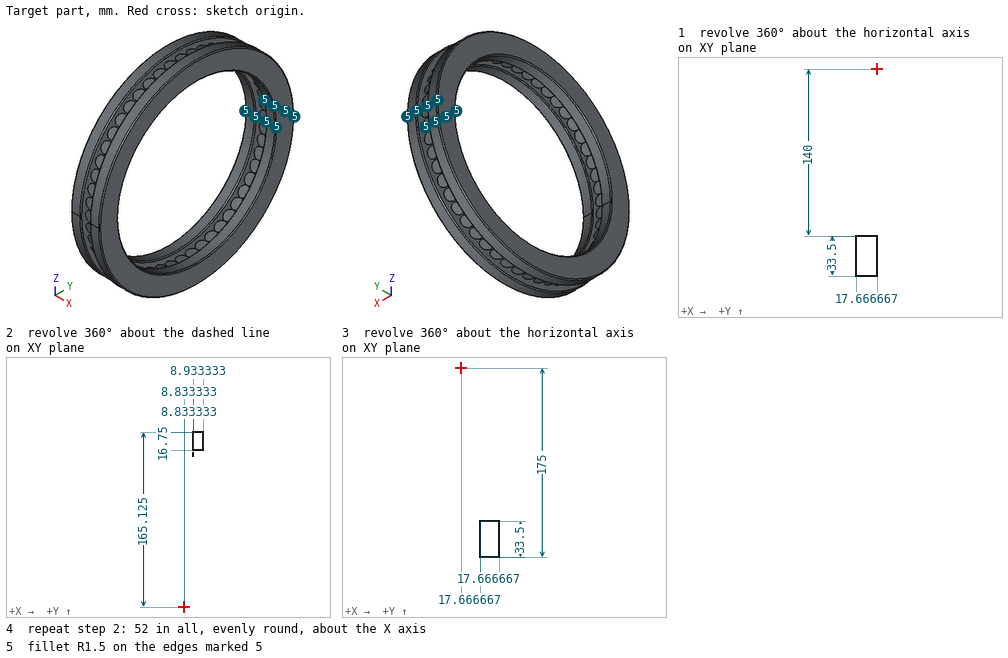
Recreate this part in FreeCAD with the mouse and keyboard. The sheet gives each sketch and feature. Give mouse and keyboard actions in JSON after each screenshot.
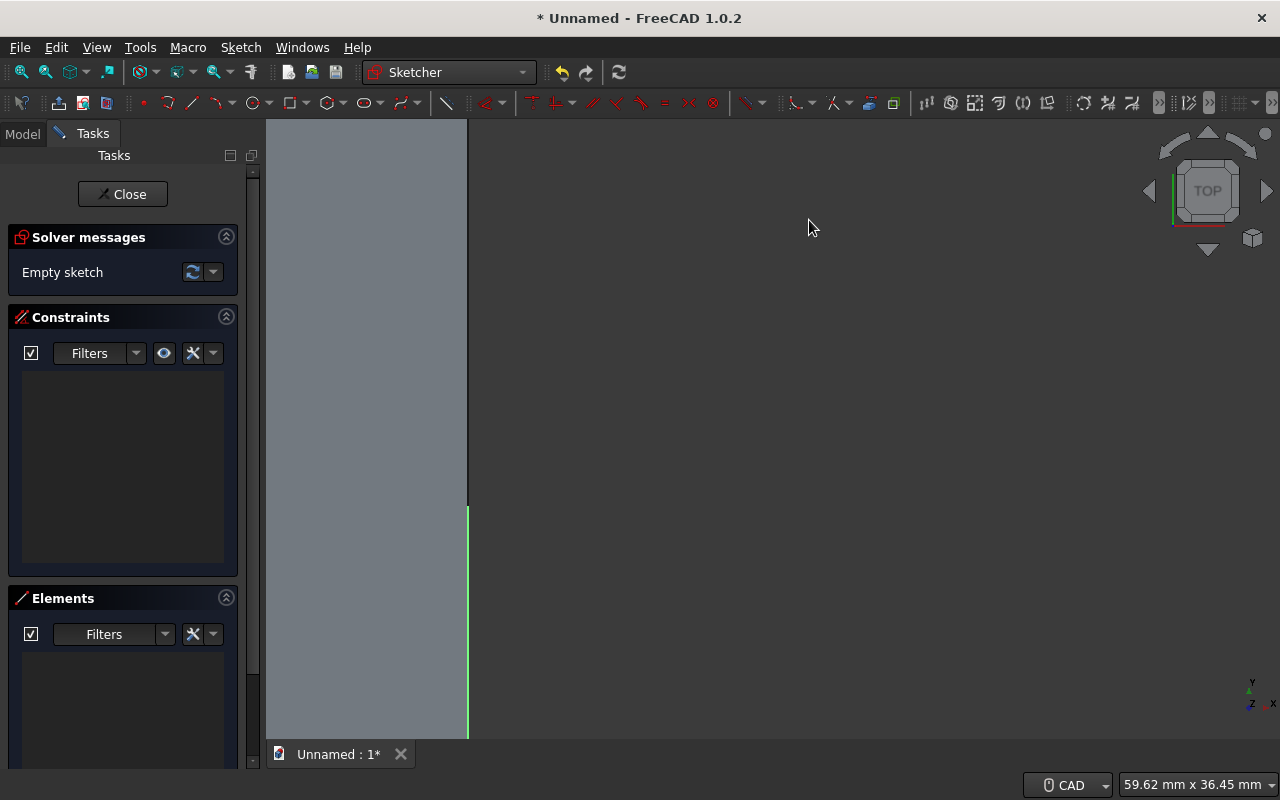
{"action": "key", "text": "g r"}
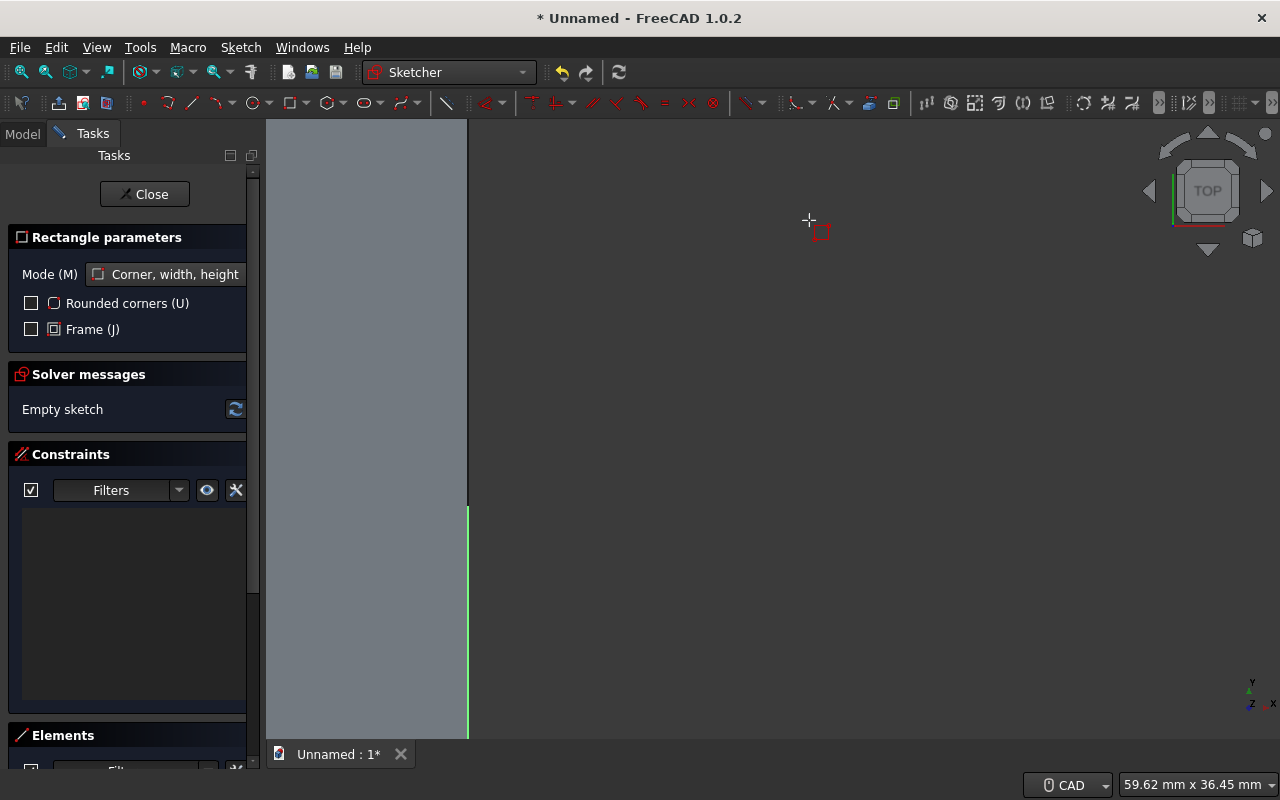
{"action": "left_click", "coordinate": [618, 222]}
{"action": "left_click", "coordinate": [770, 506]}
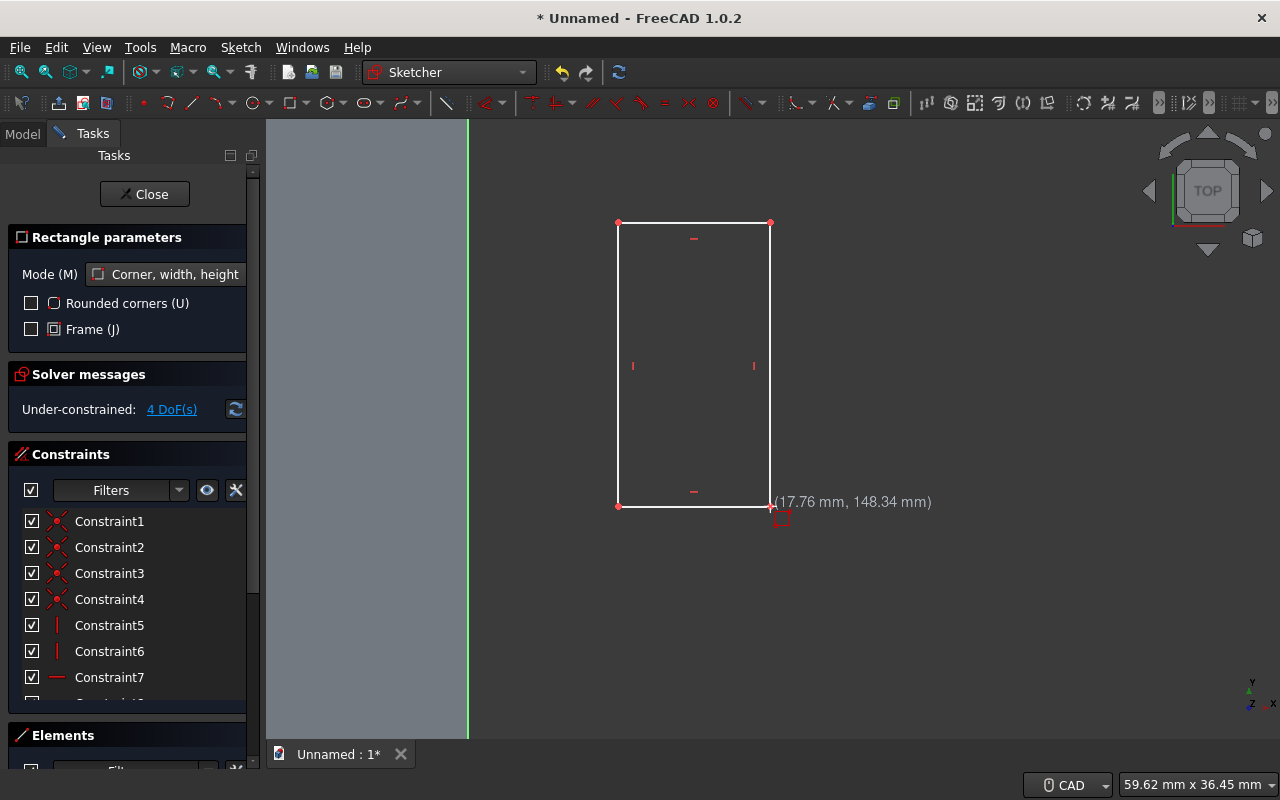
{"action": "left_click", "coordinate": [192, 104]}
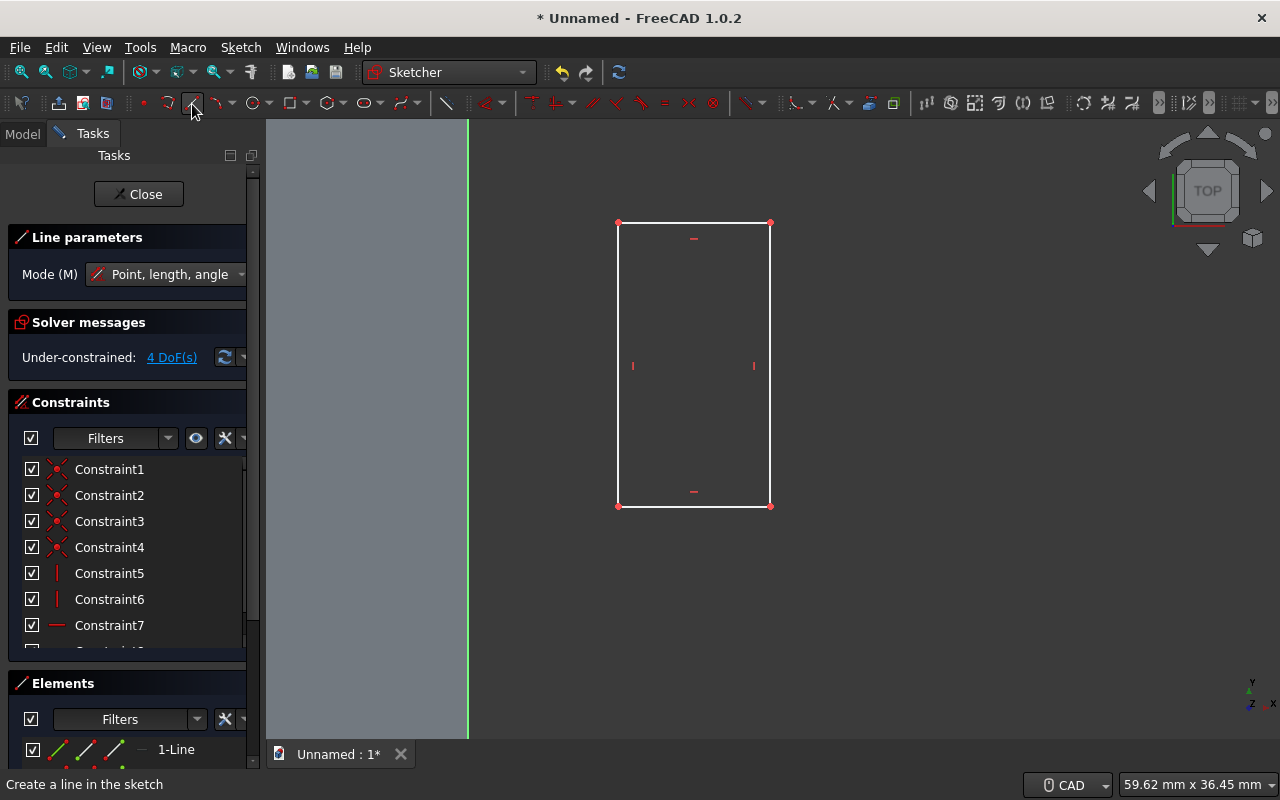
{"action": "left_click", "coordinate": [618, 535]}
{"action": "left_click", "coordinate": [618, 620]}
{"action": "key", "text": "Escape"}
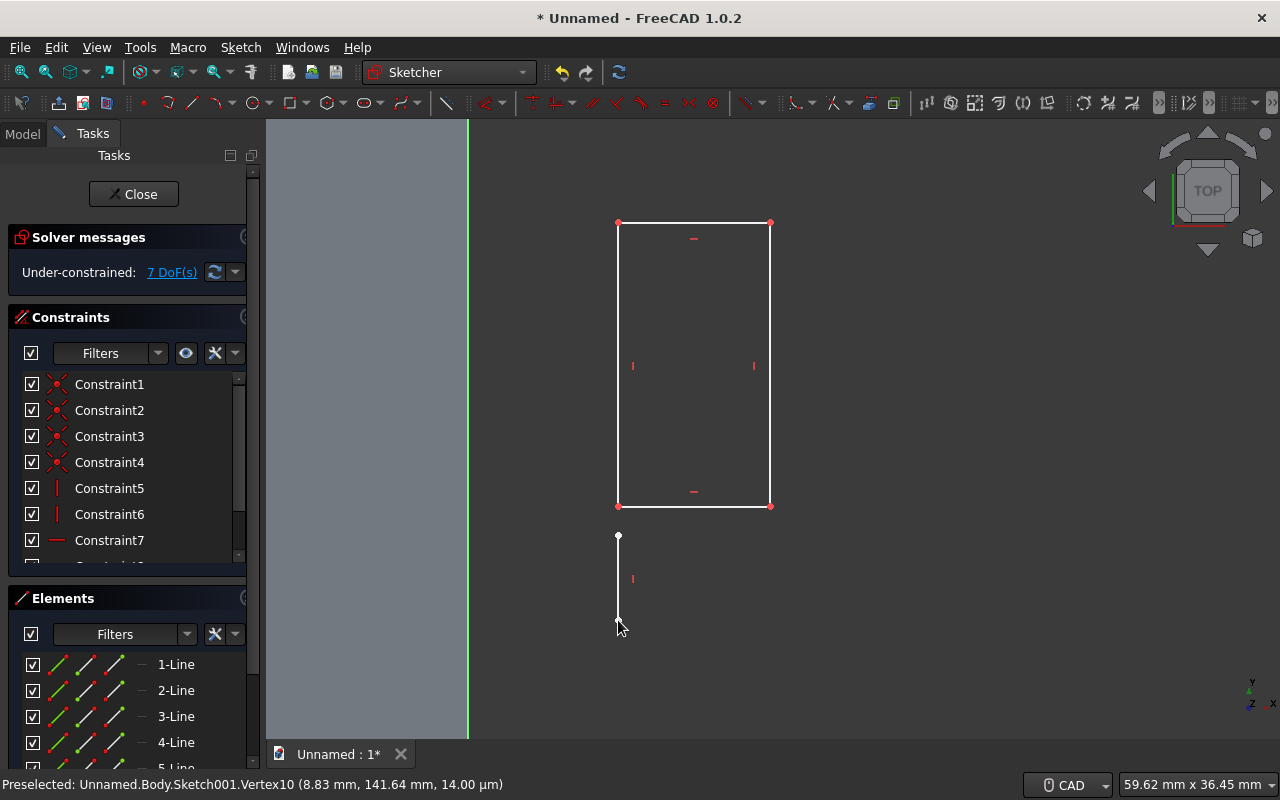
{"action": "left_click", "coordinate": [618, 561]}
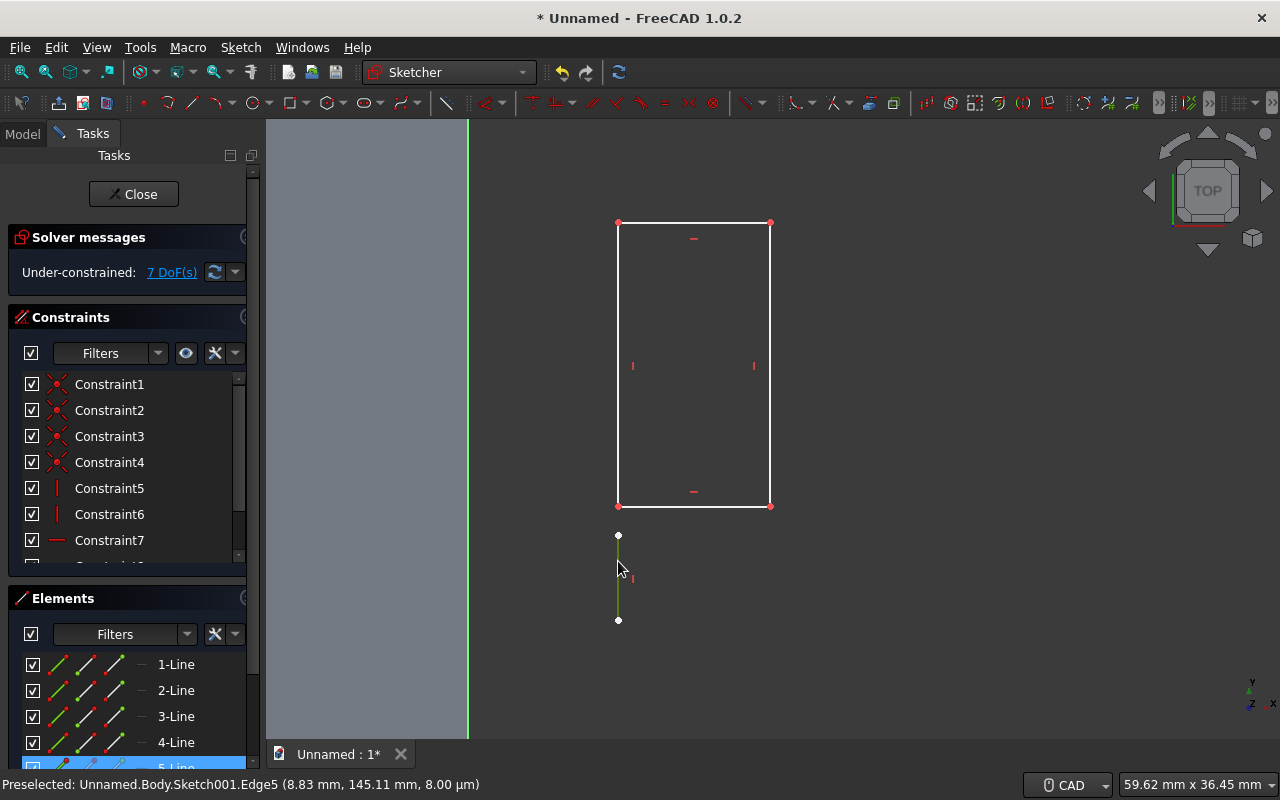
{"action": "left_click", "coordinate": [448, 104]}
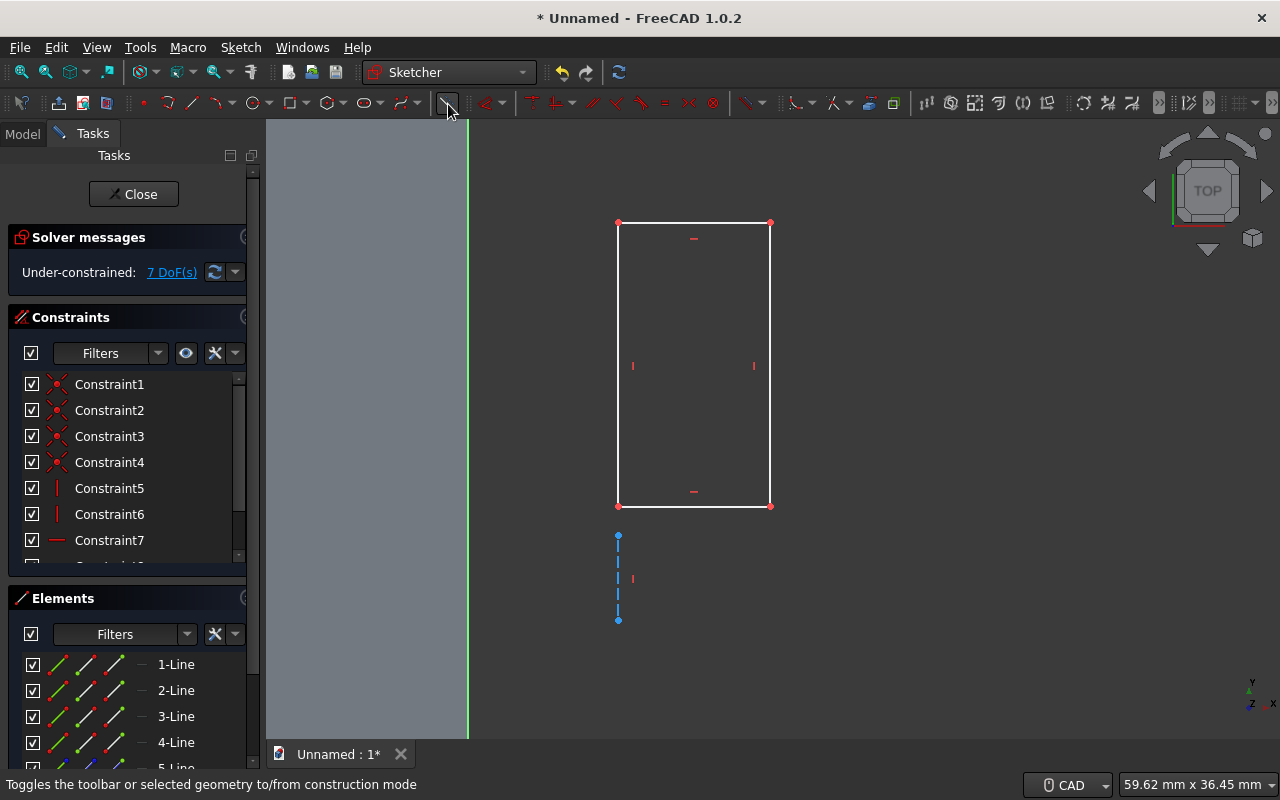
{"action": "left_click", "coordinate": [486, 104]}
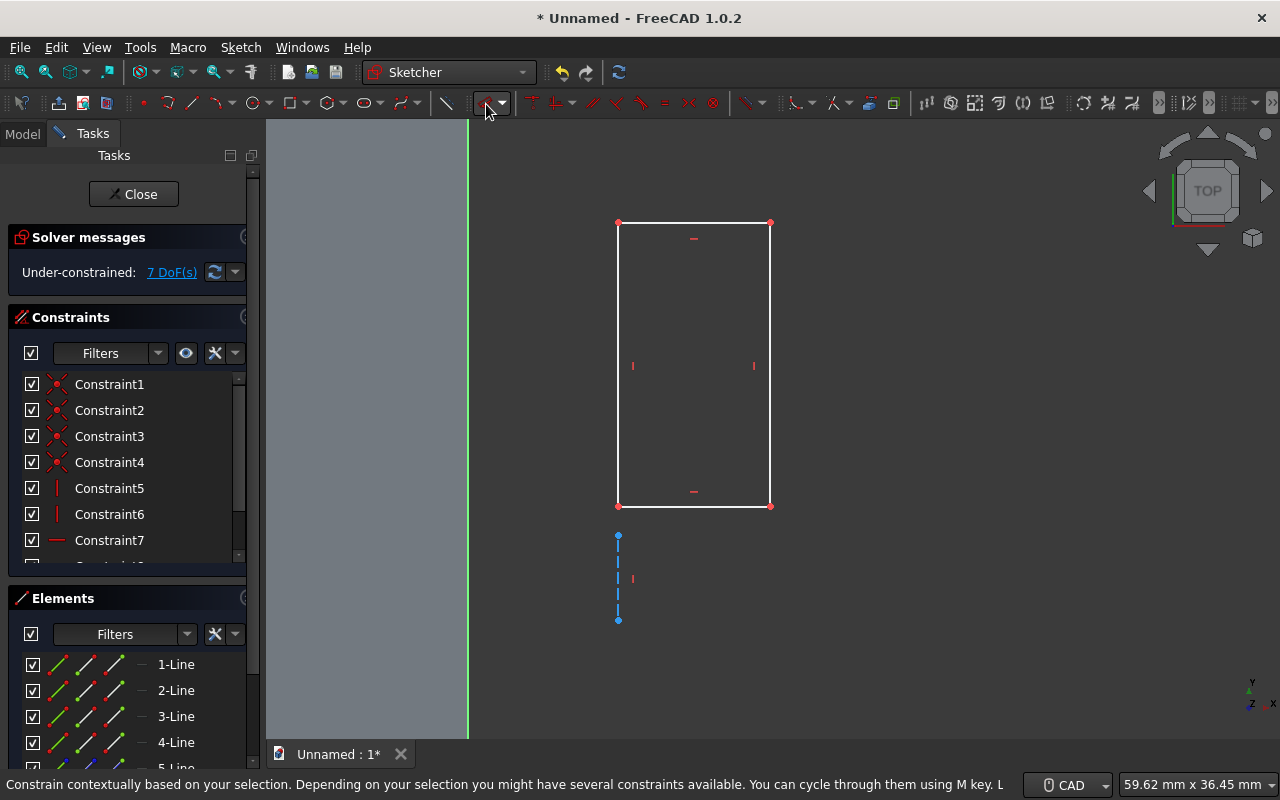
{"action": "left_click", "coordinate": [618, 308]}
{"action": "left_click", "coordinate": [584, 365]}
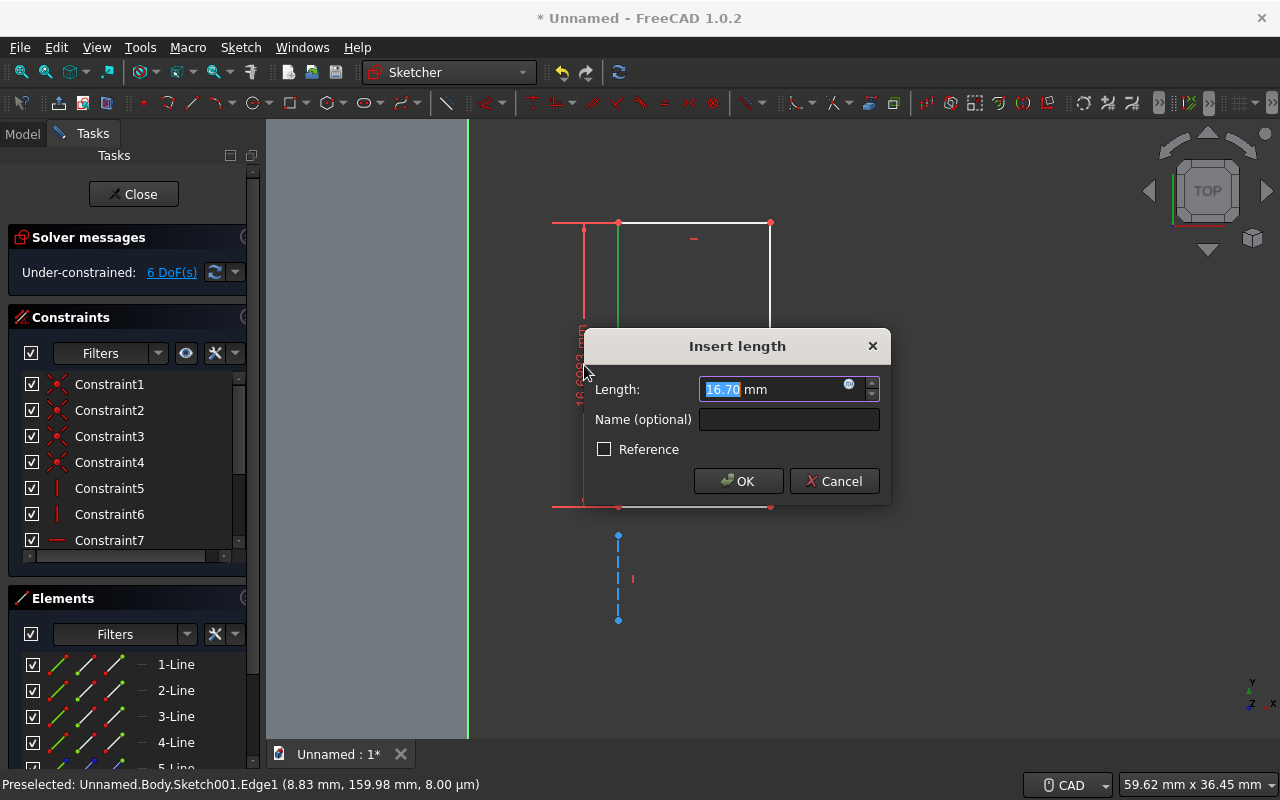
{"action": "type", "text": "16.75"}
{"action": "key", "text": "Return"}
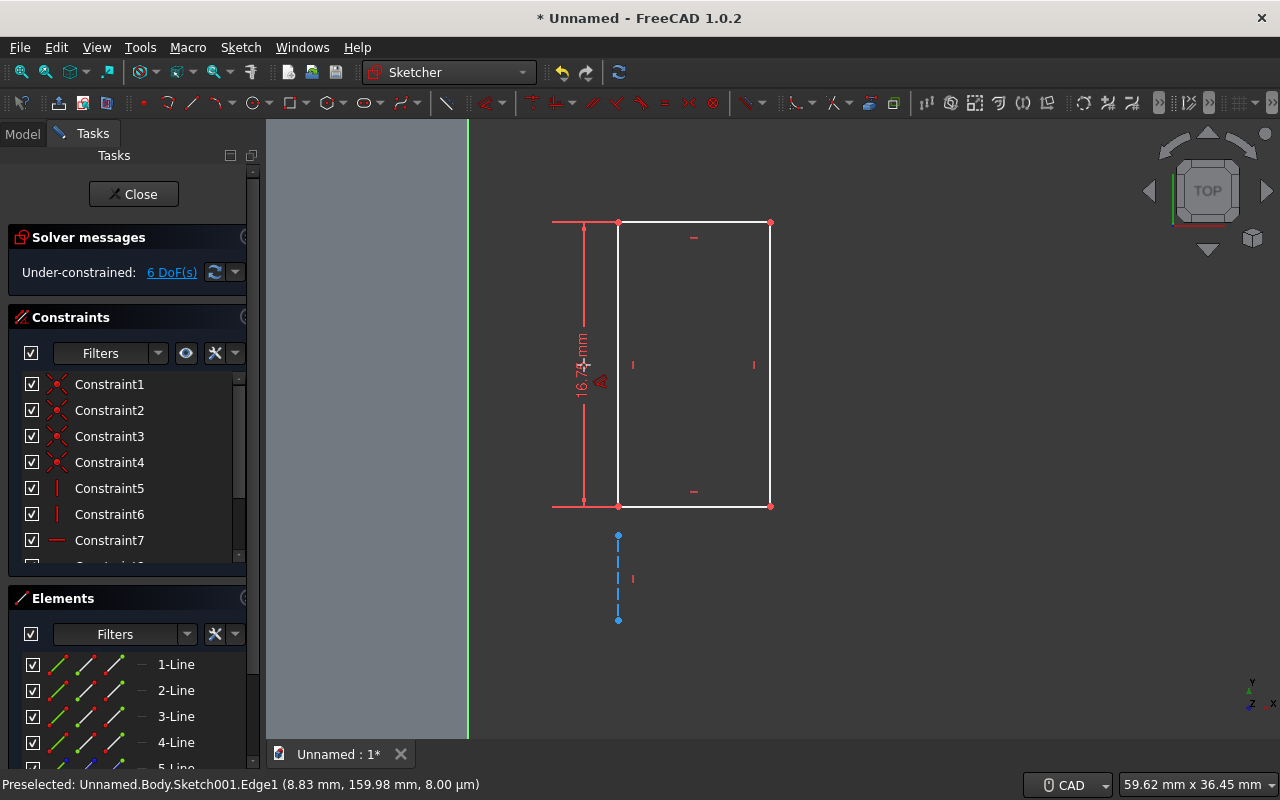
{"action": "left_click", "coordinate": [664, 507]}
{"action": "left_click", "coordinate": [694, 541]}